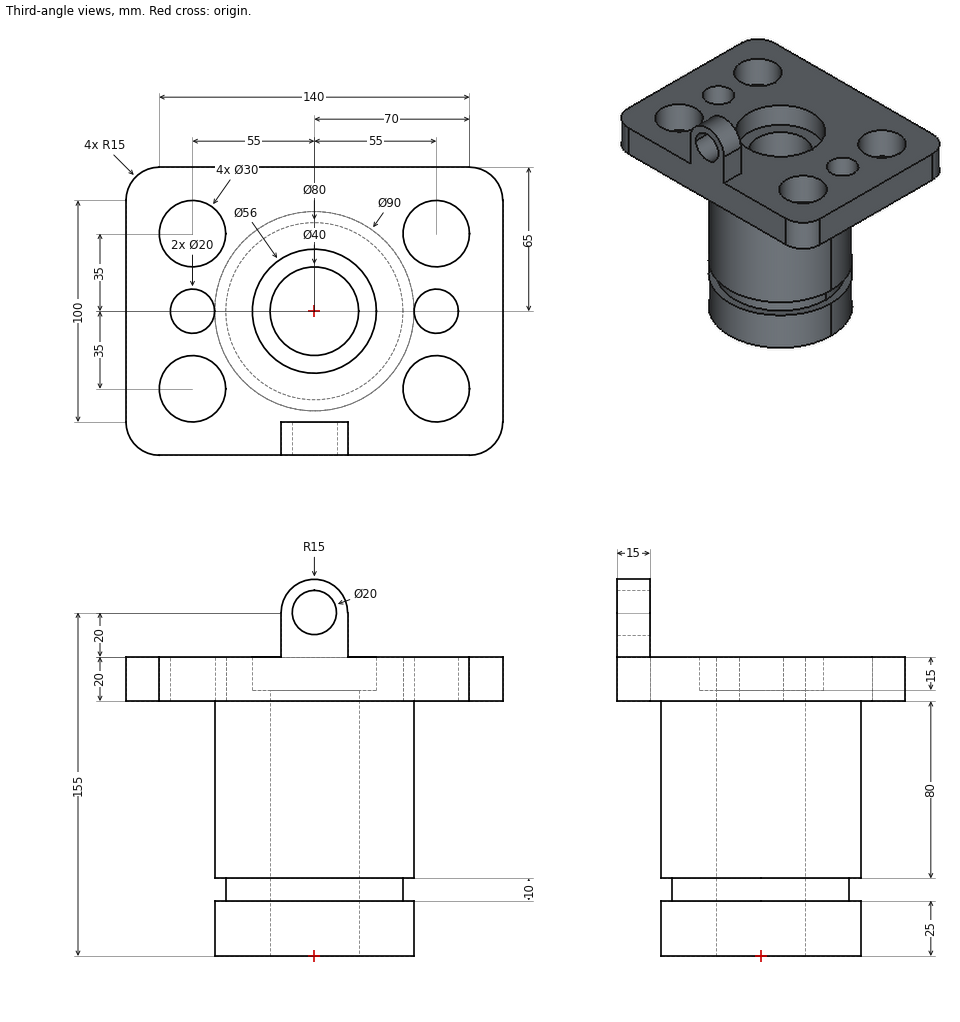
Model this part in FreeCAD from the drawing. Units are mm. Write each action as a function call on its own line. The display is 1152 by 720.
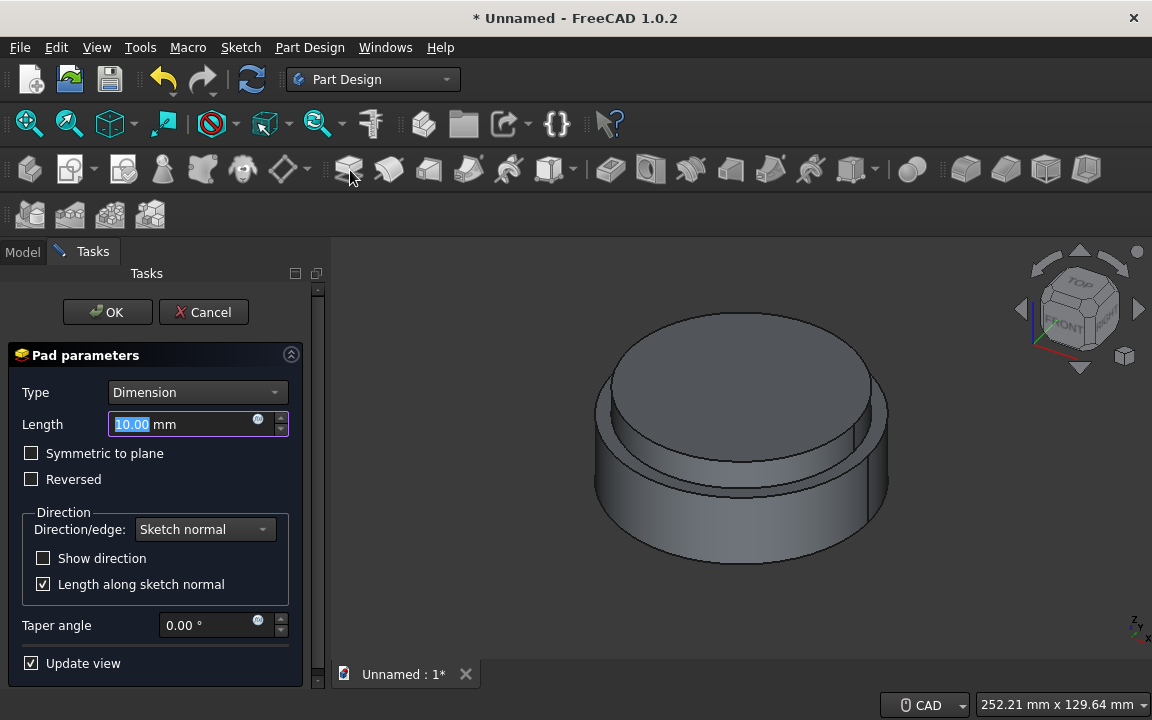
text(10)
key(Tab)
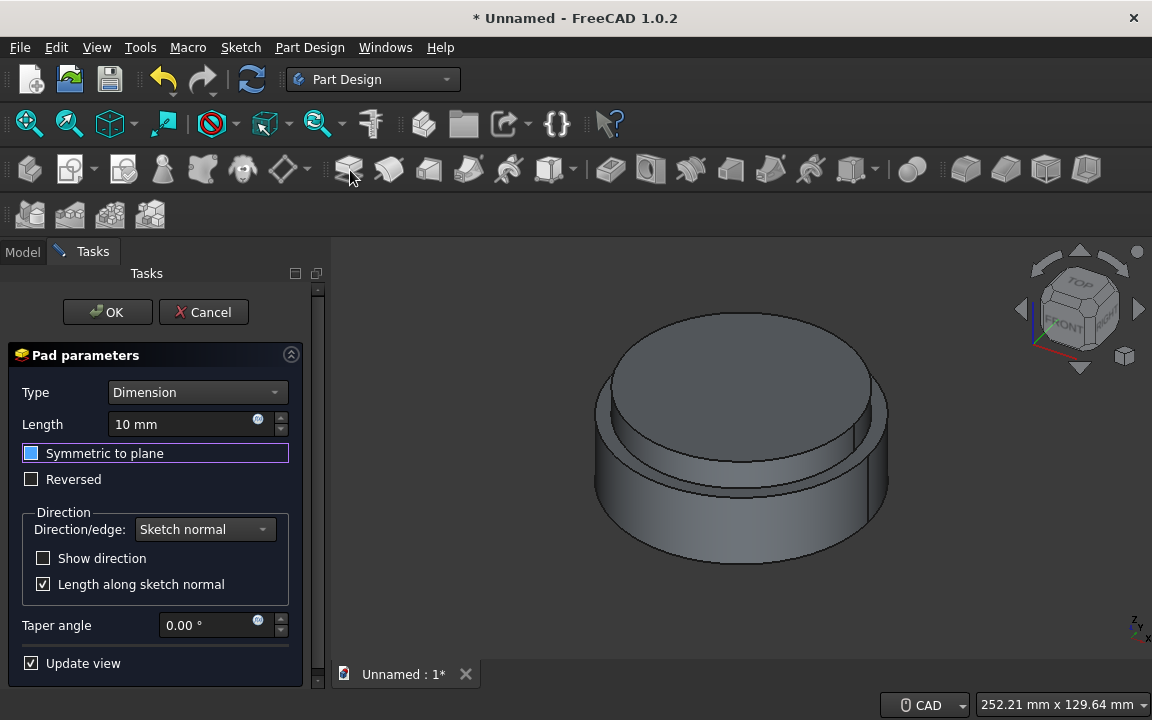
click(108, 312)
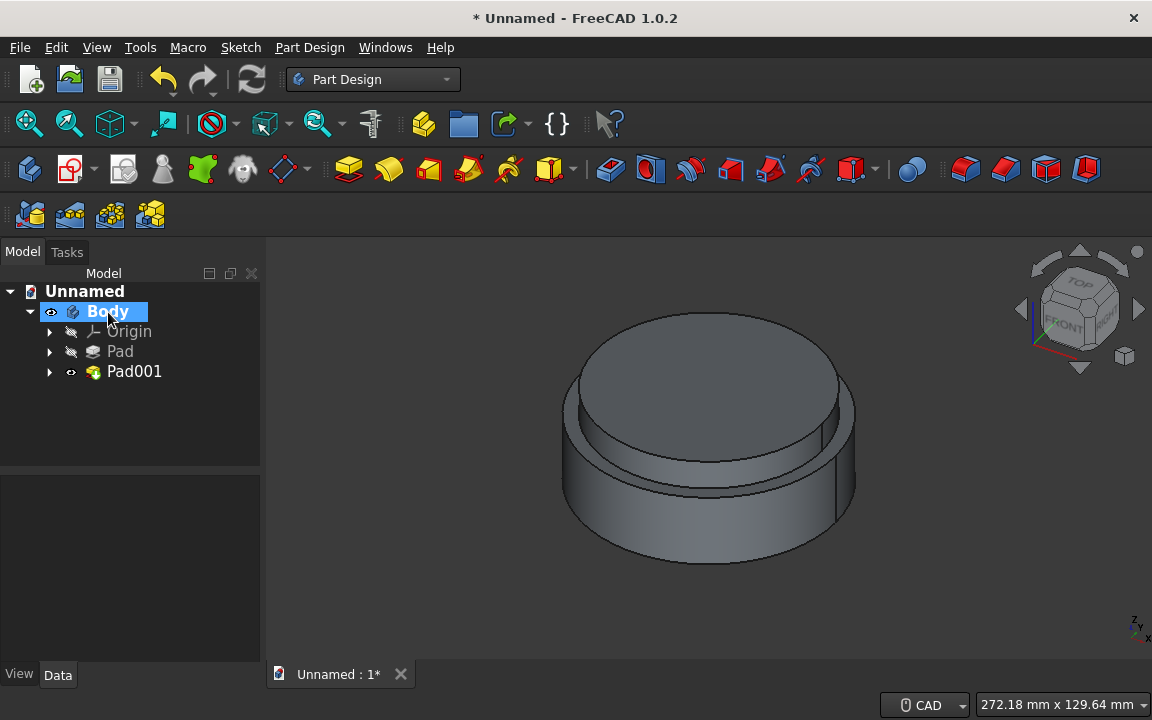
click(709, 386)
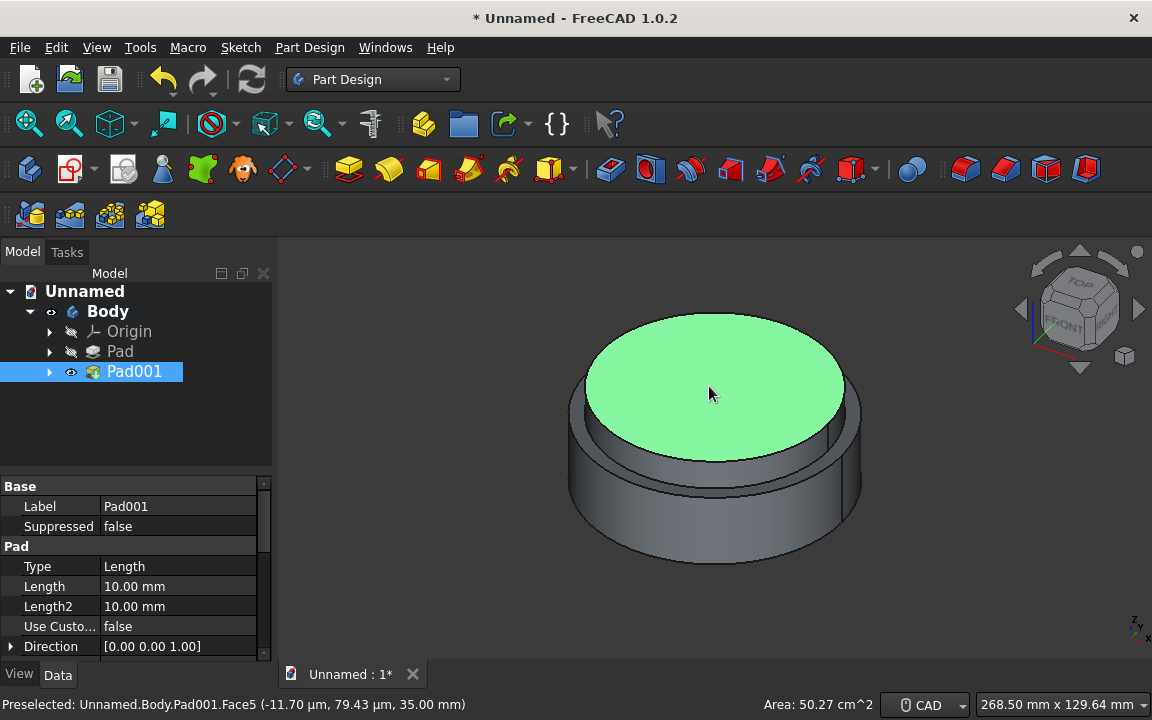
click(70, 170)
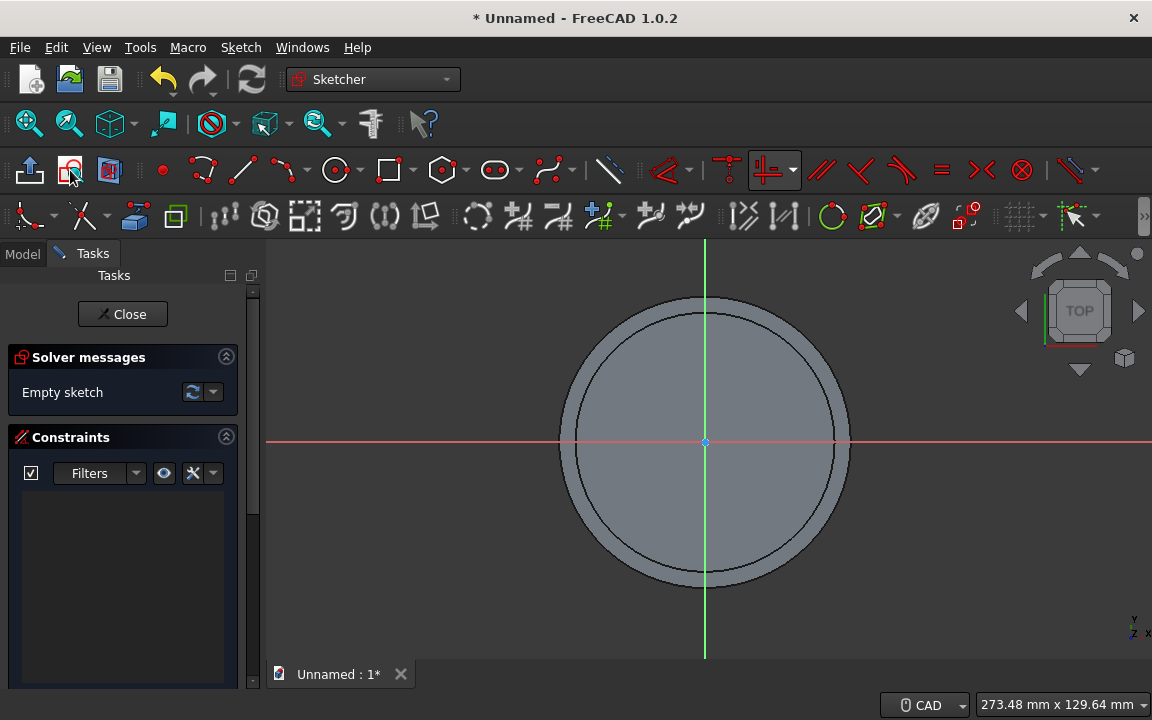
click(336, 170)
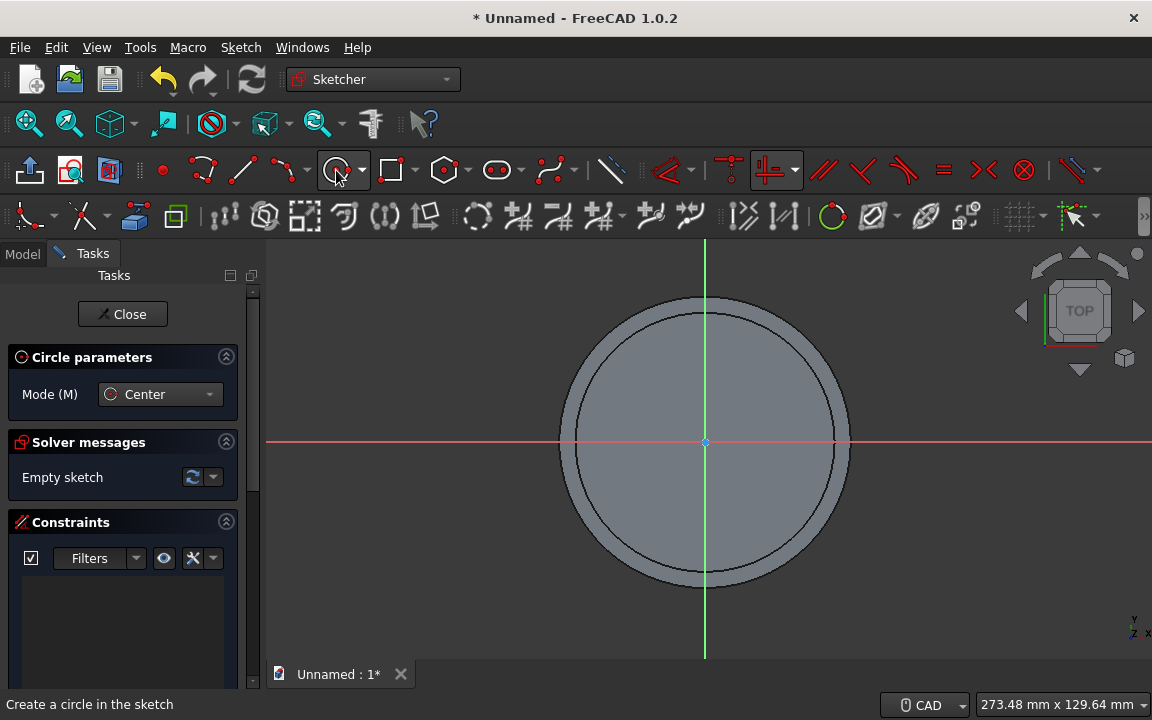
click(705, 442)
click(808, 339)
key(Escape)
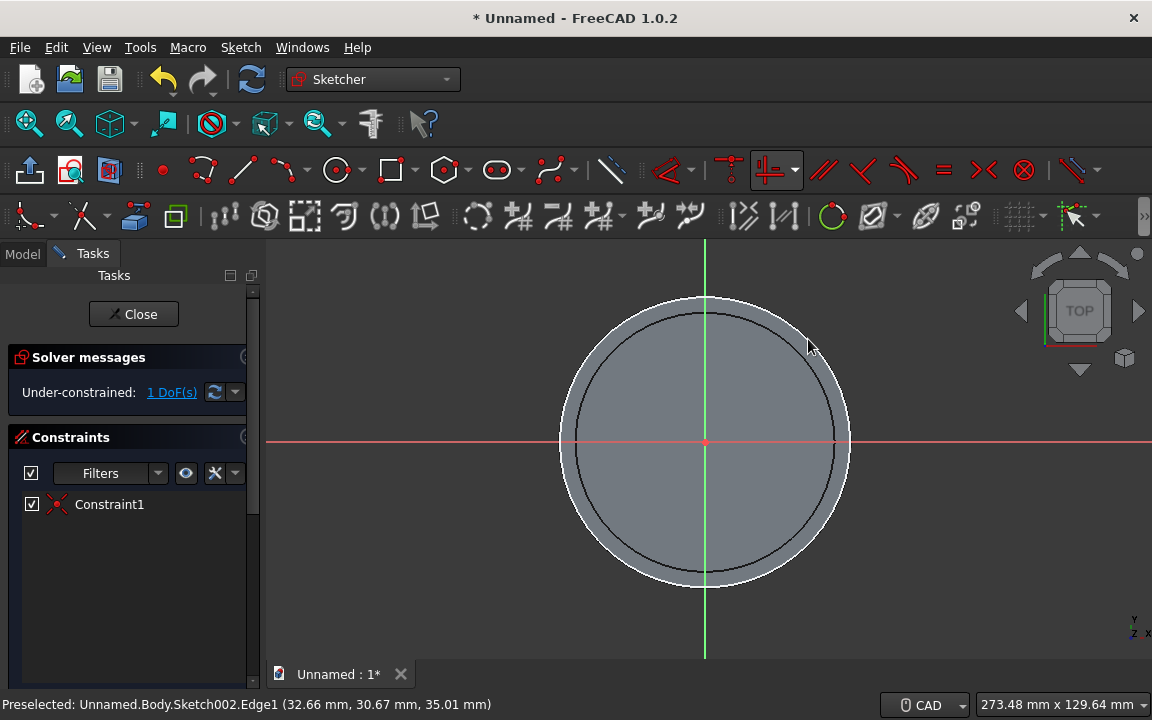
click(666, 170)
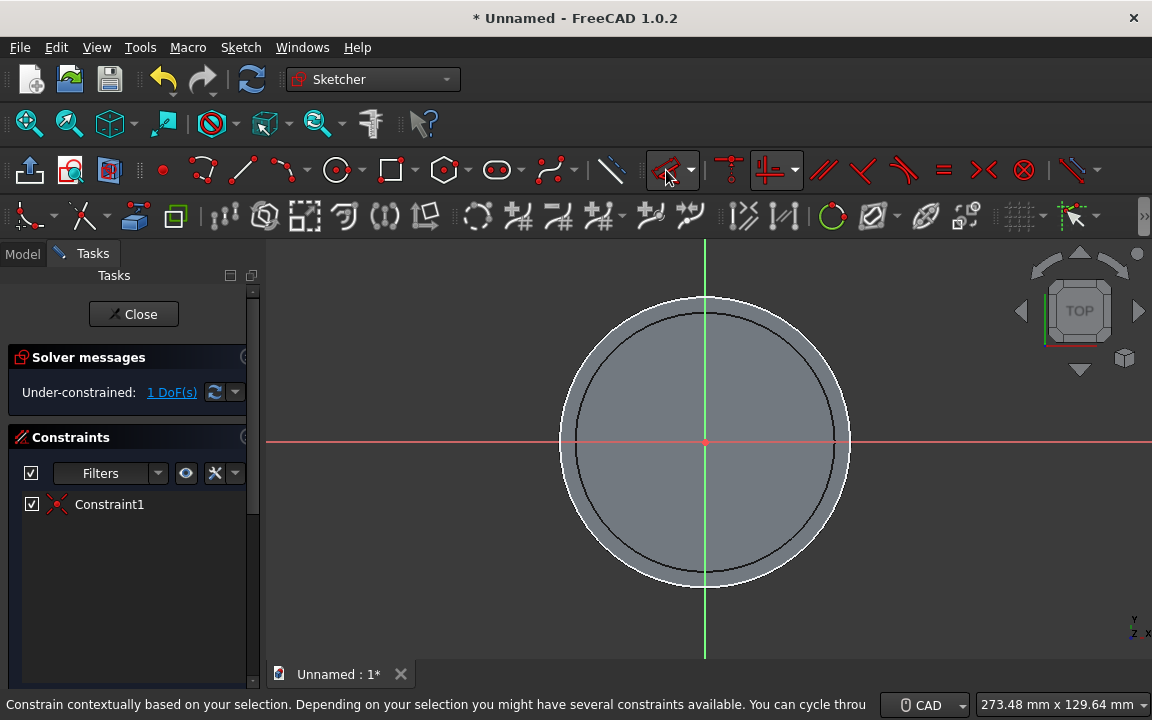
click(807, 339)
click(829, 316)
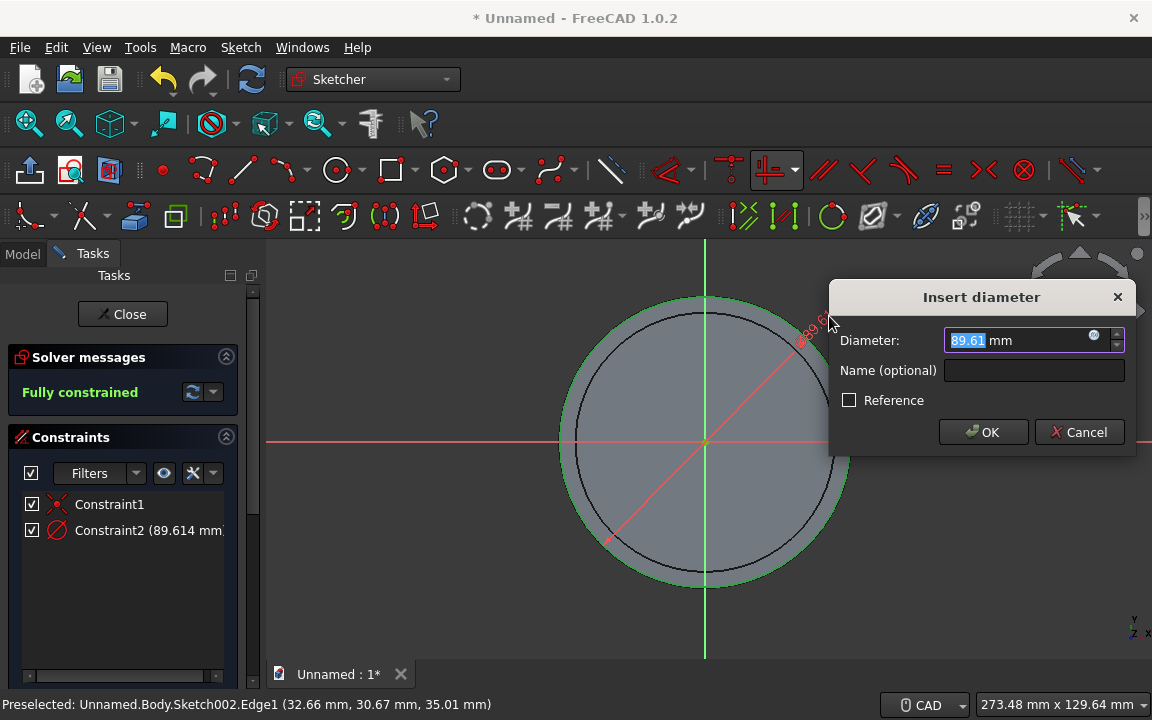
text(90)
key(Return)
key(Escape)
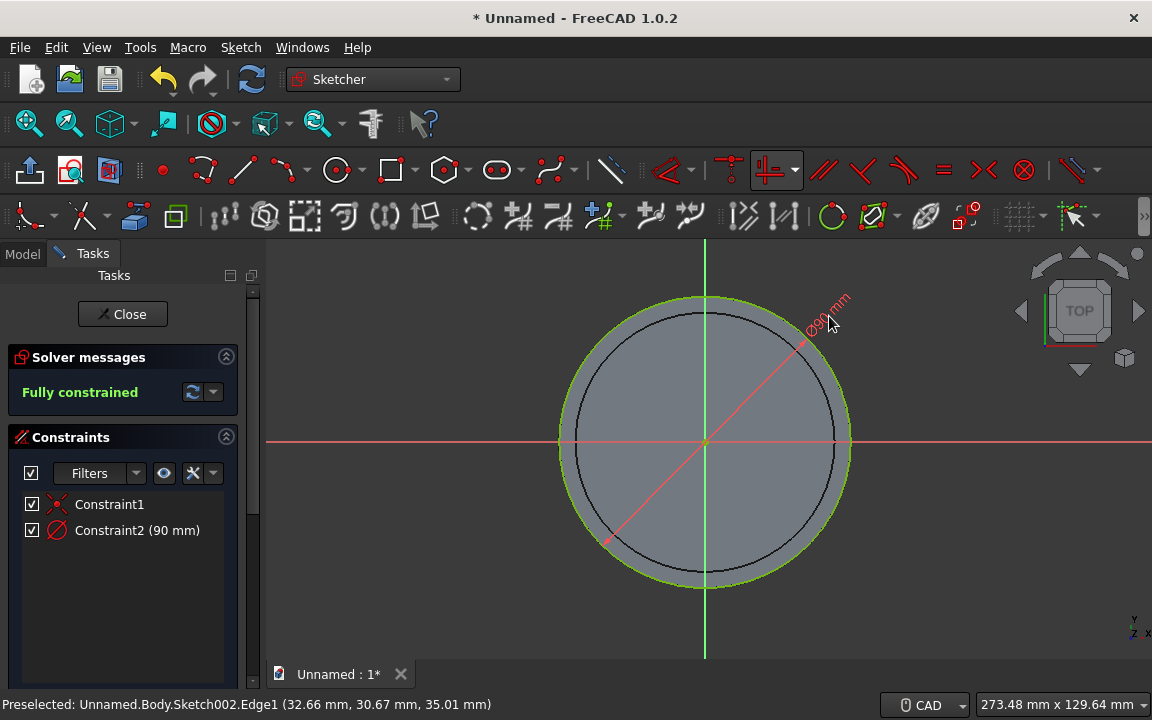
click(123, 314)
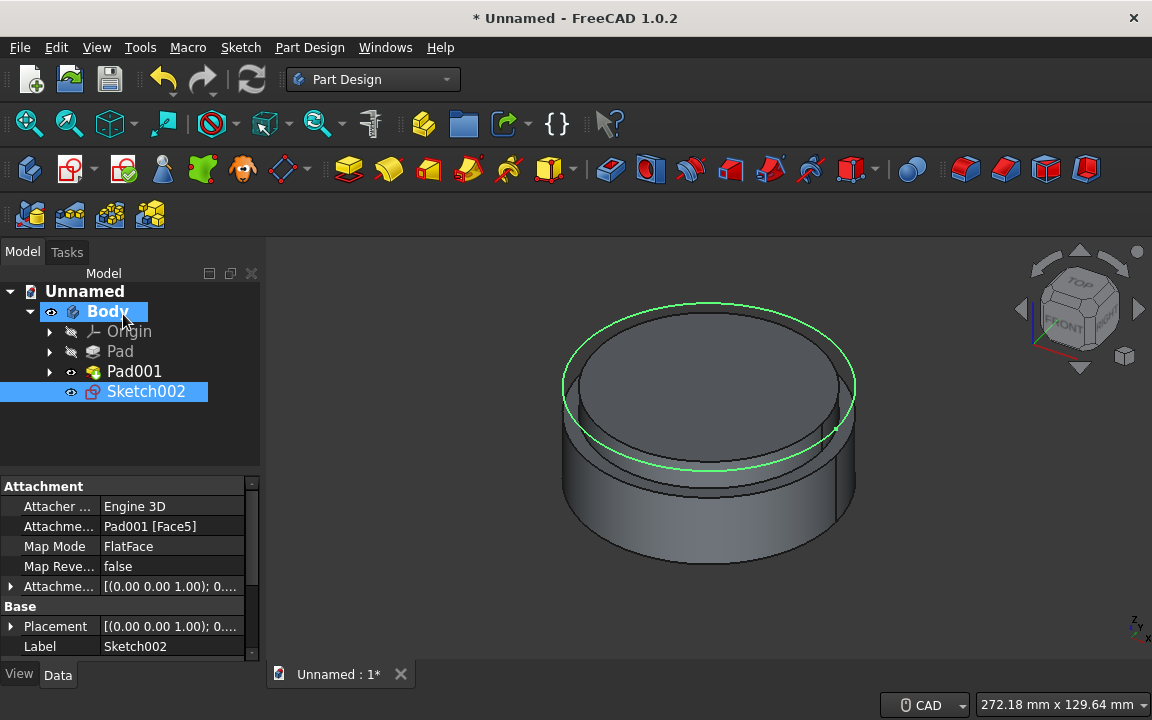
click(350, 170)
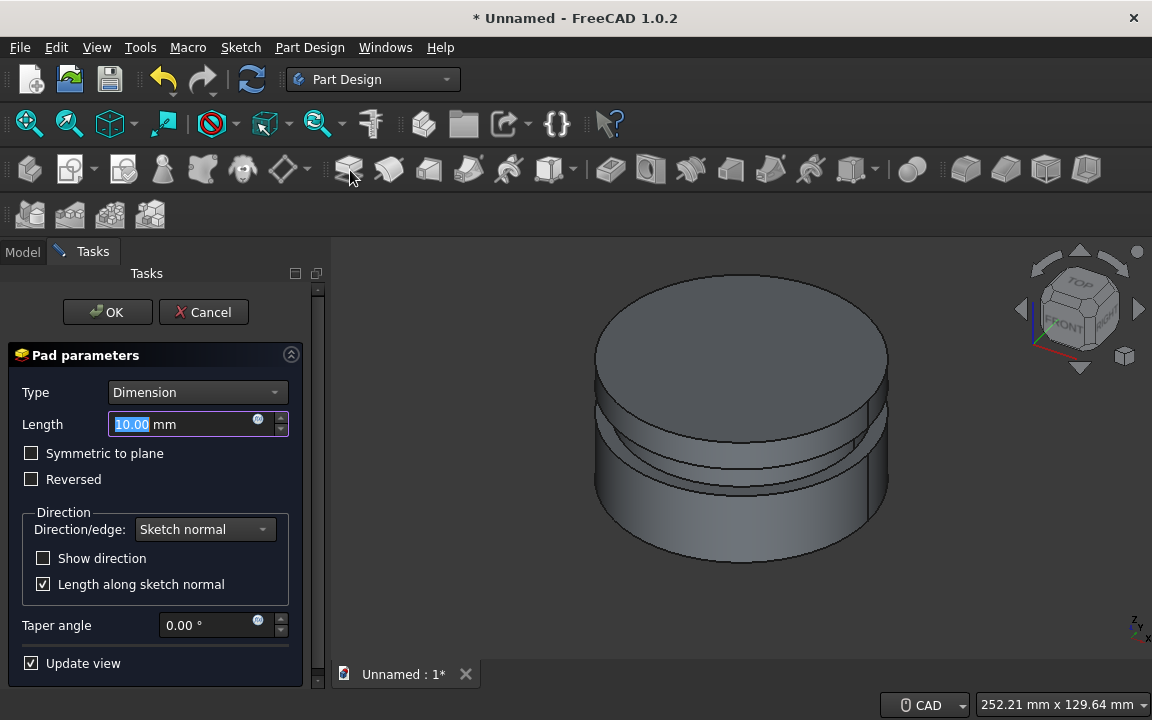
text(80)
key(Tab)